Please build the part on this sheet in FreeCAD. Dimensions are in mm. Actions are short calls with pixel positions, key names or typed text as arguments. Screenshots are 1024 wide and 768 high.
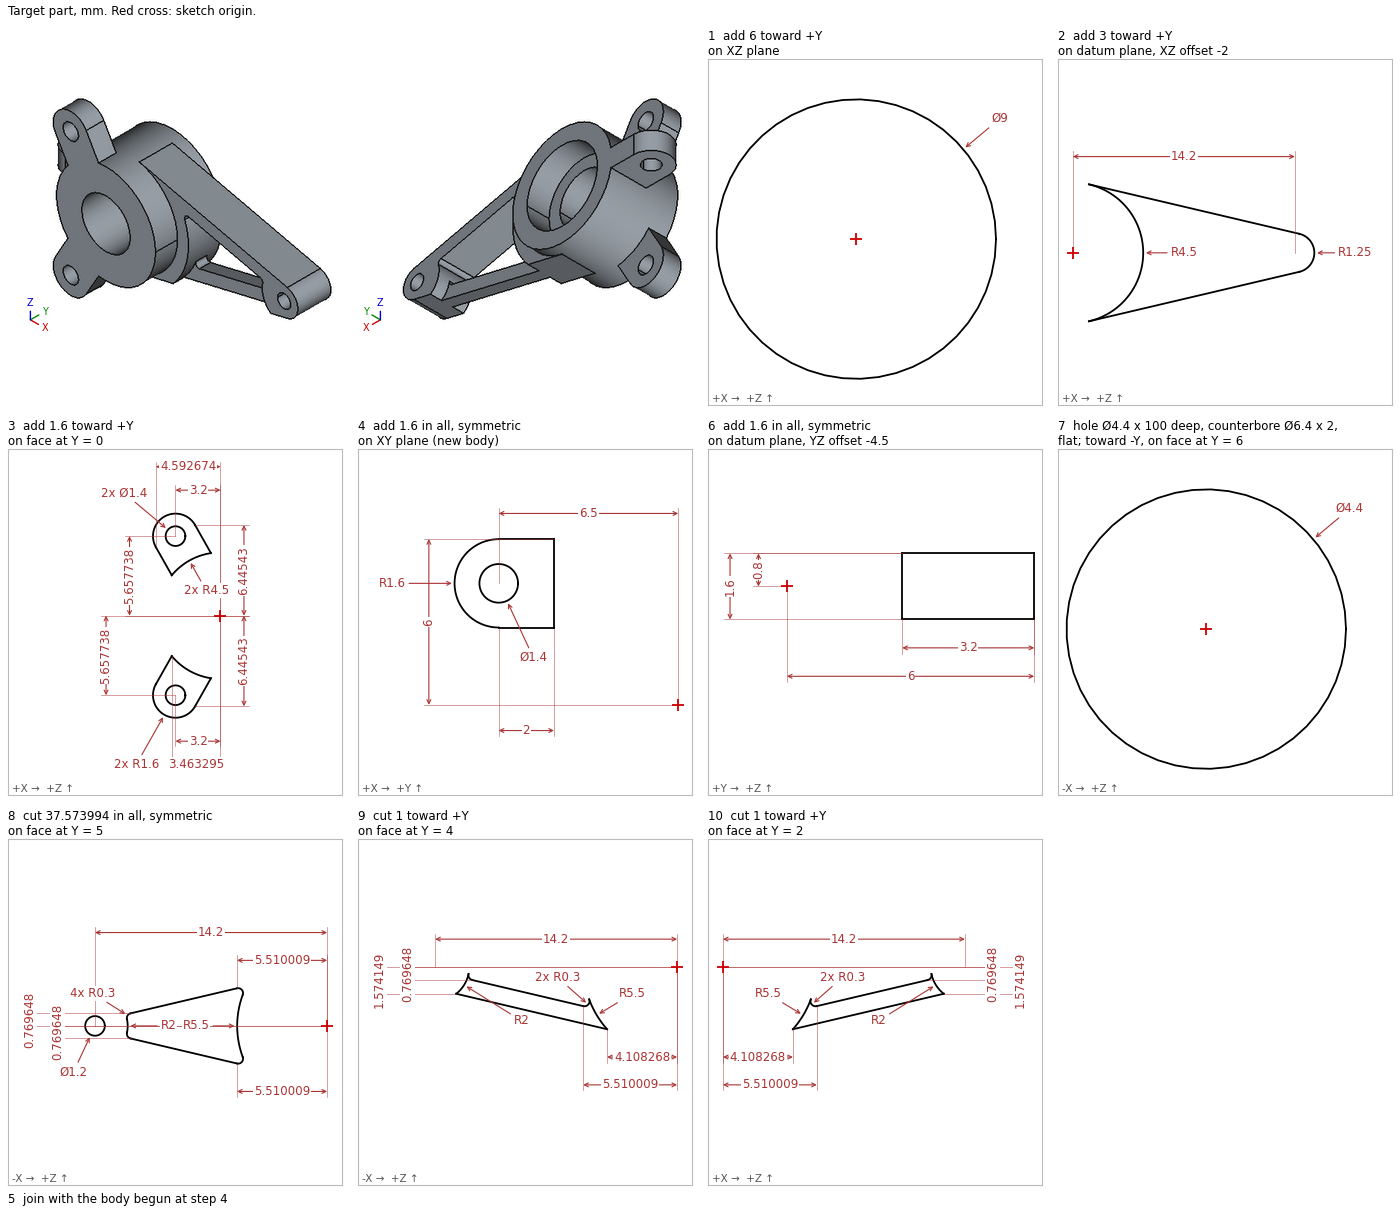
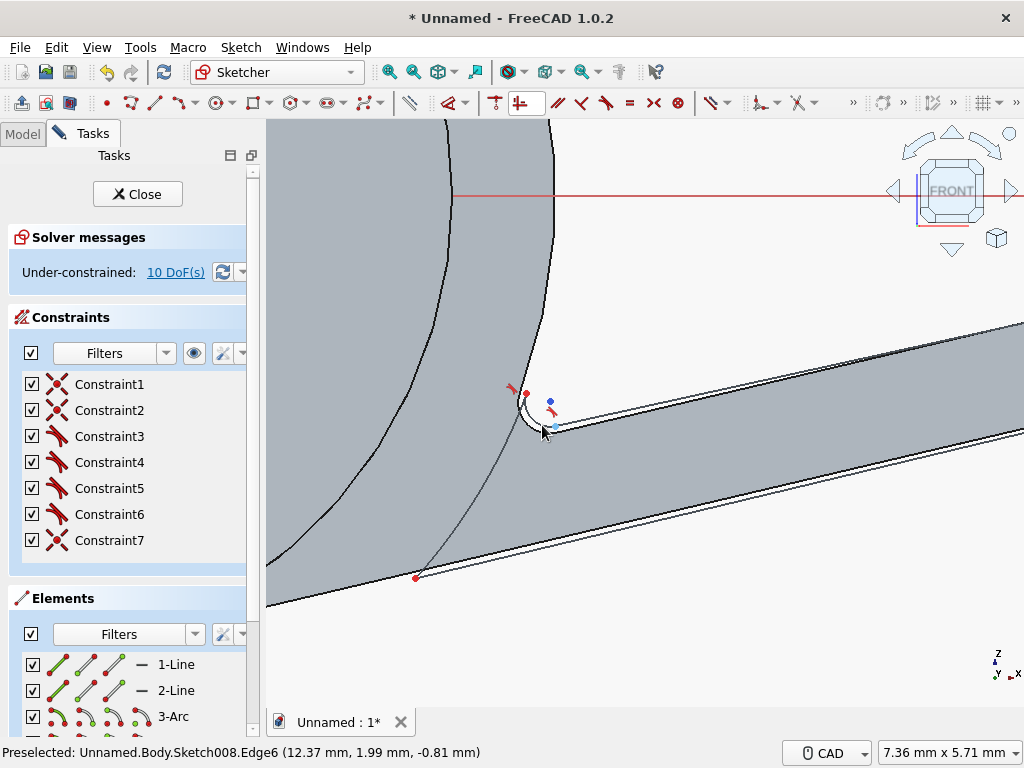
click(540, 425)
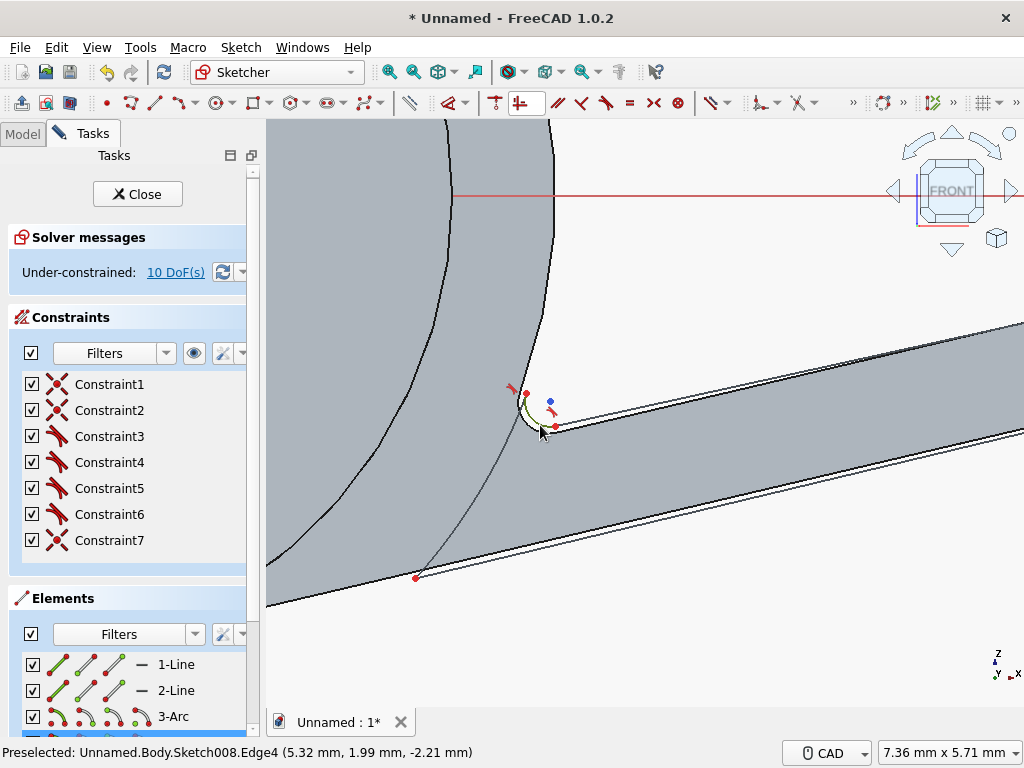
scroll(542, 425, down, 6)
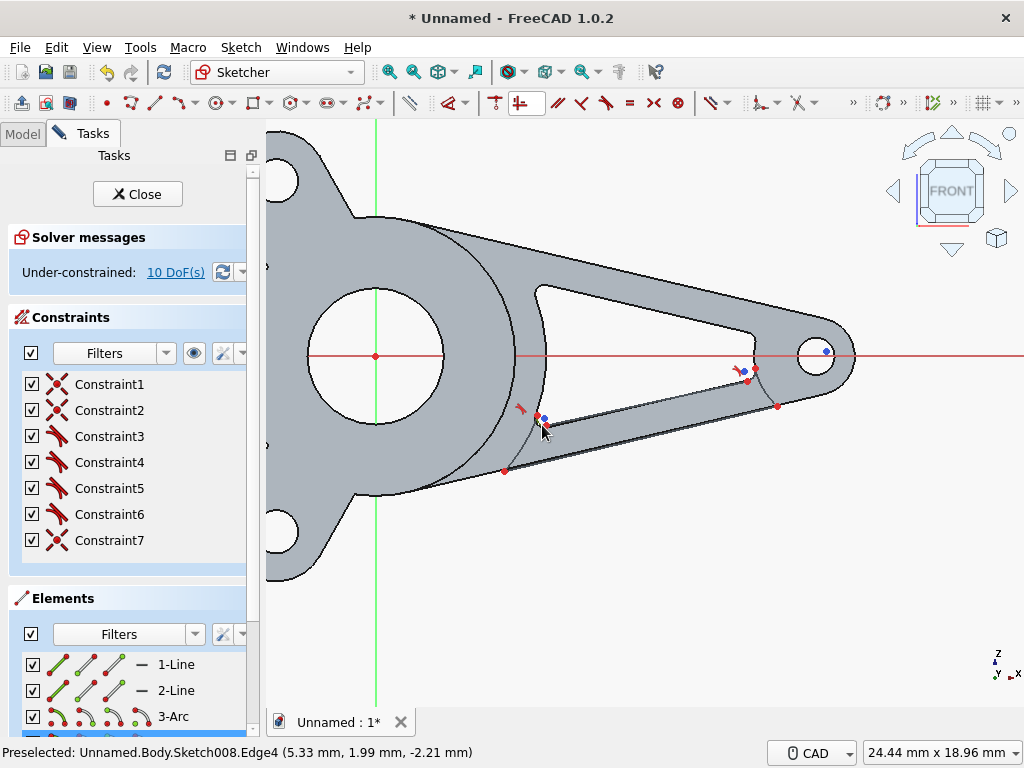
scroll(752, 379, up, 6)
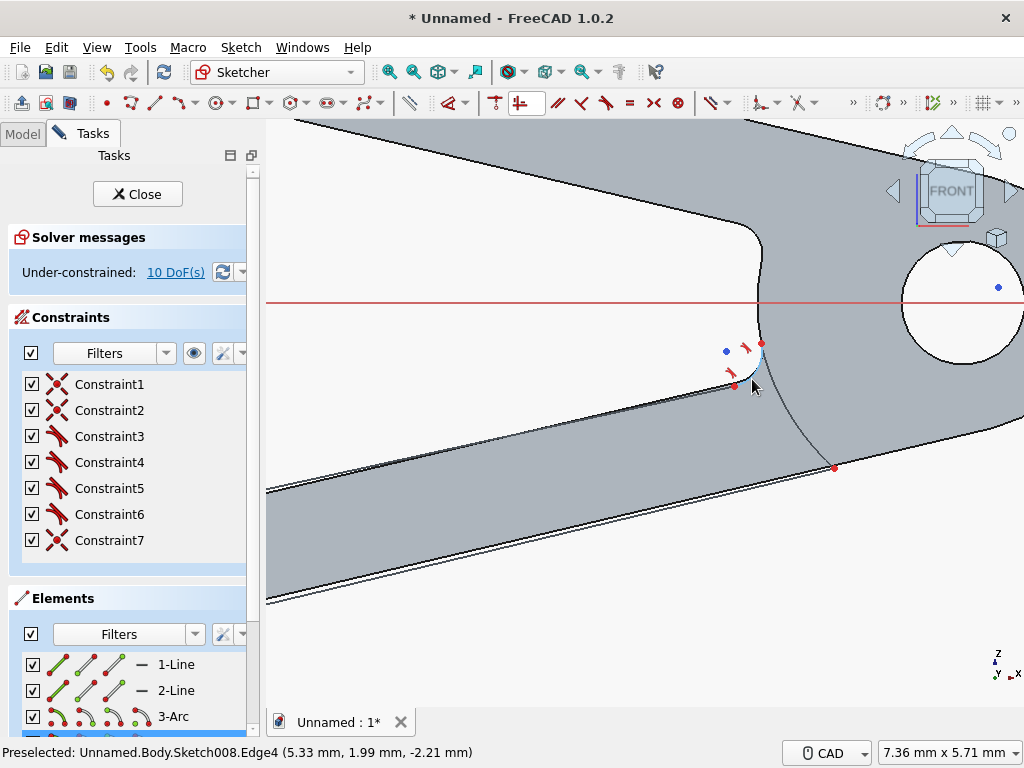
click(749, 379)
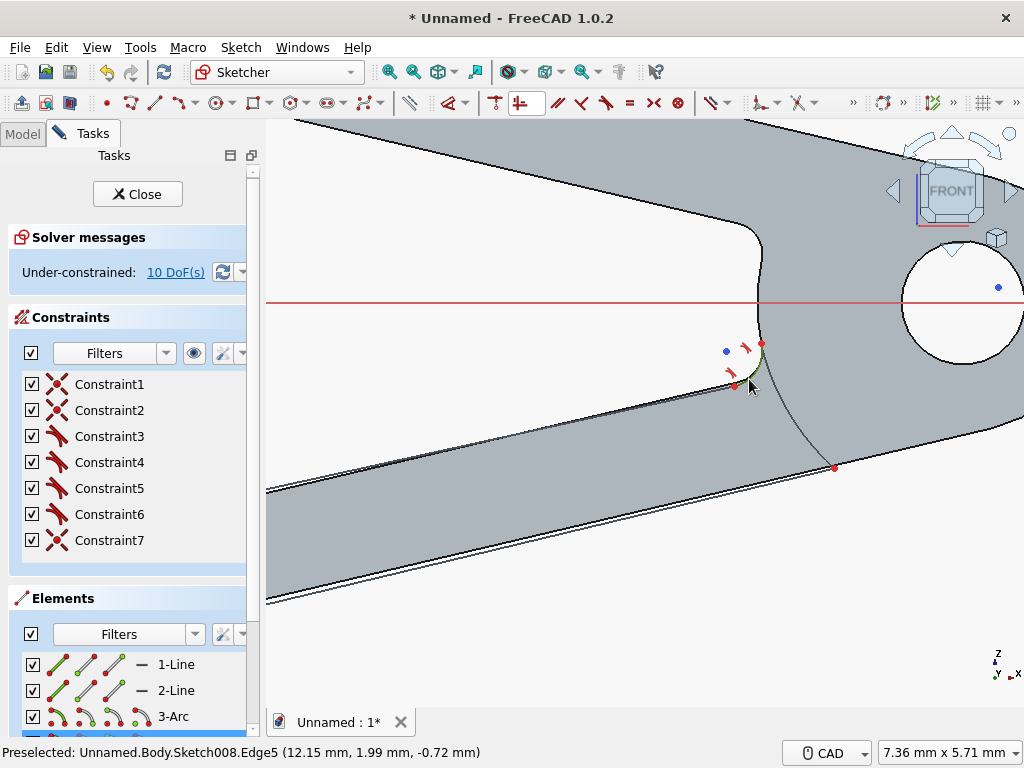
key(e)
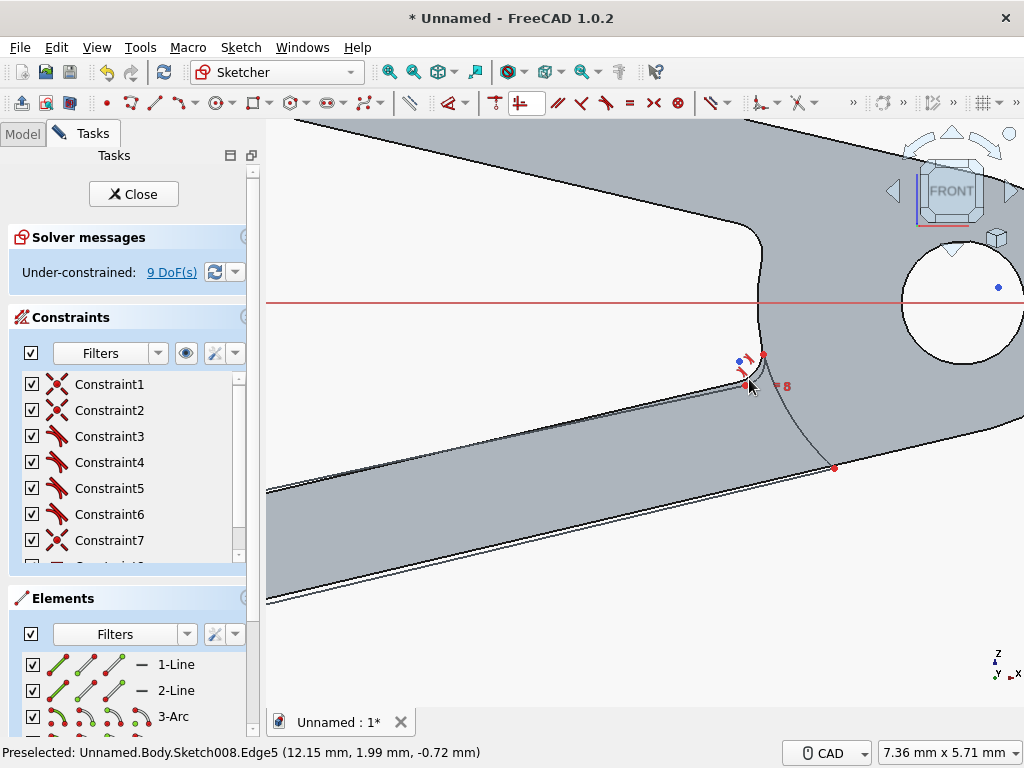
scroll(752, 379, down, 6)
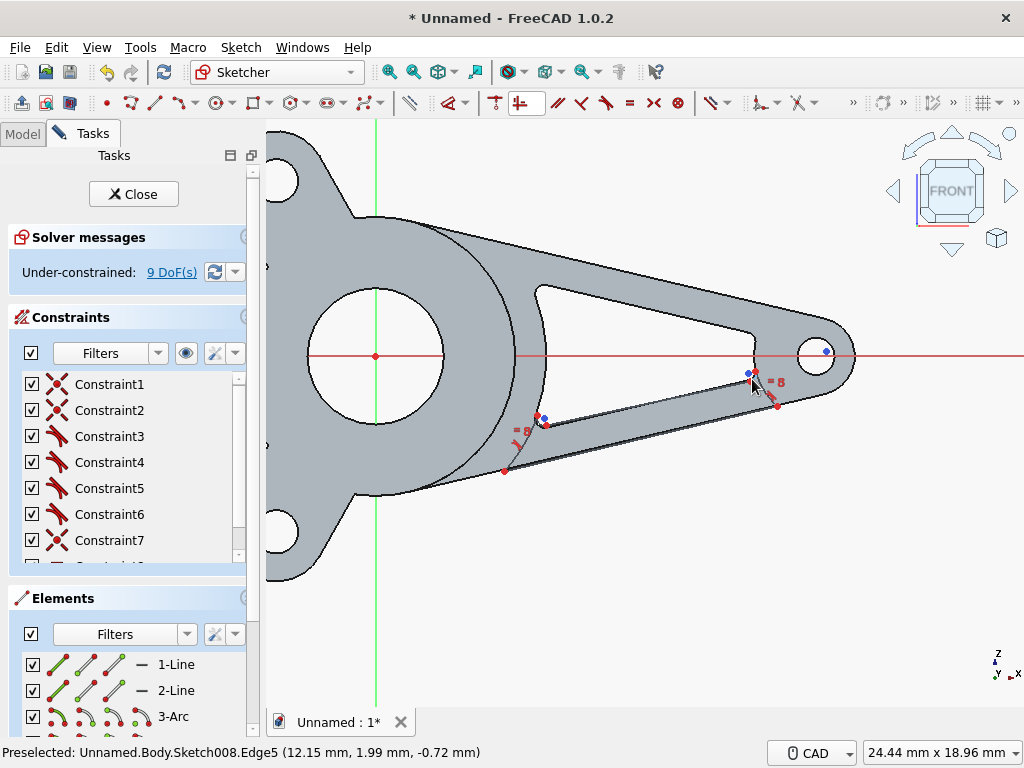
click(827, 352)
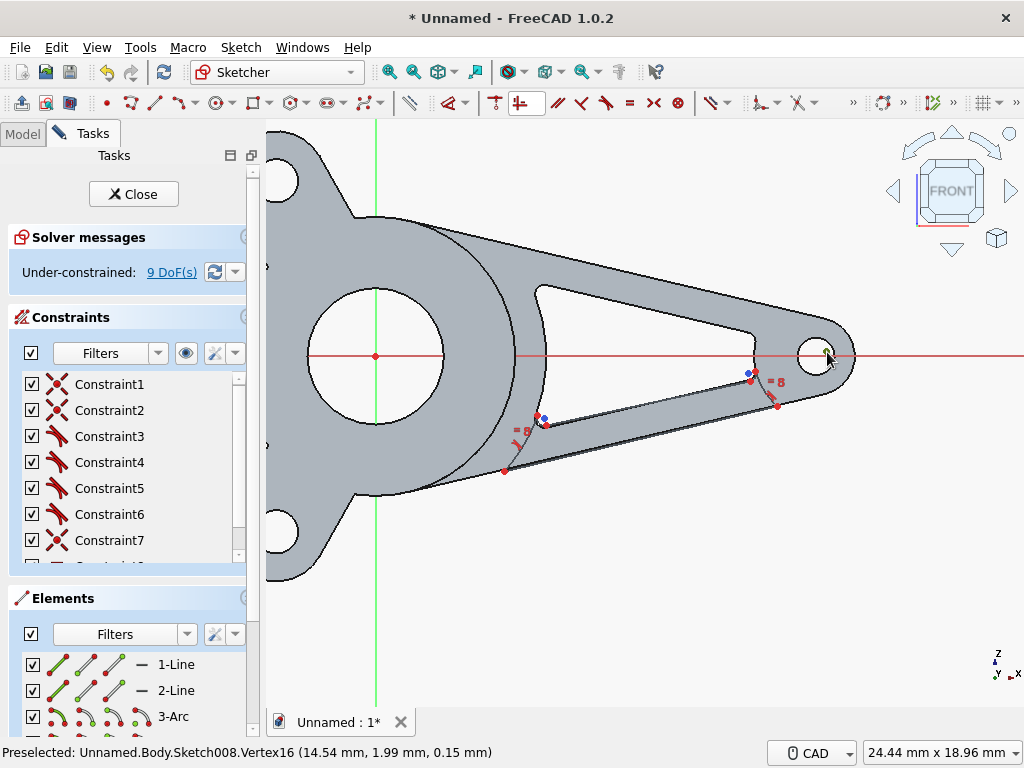
click(334, 356)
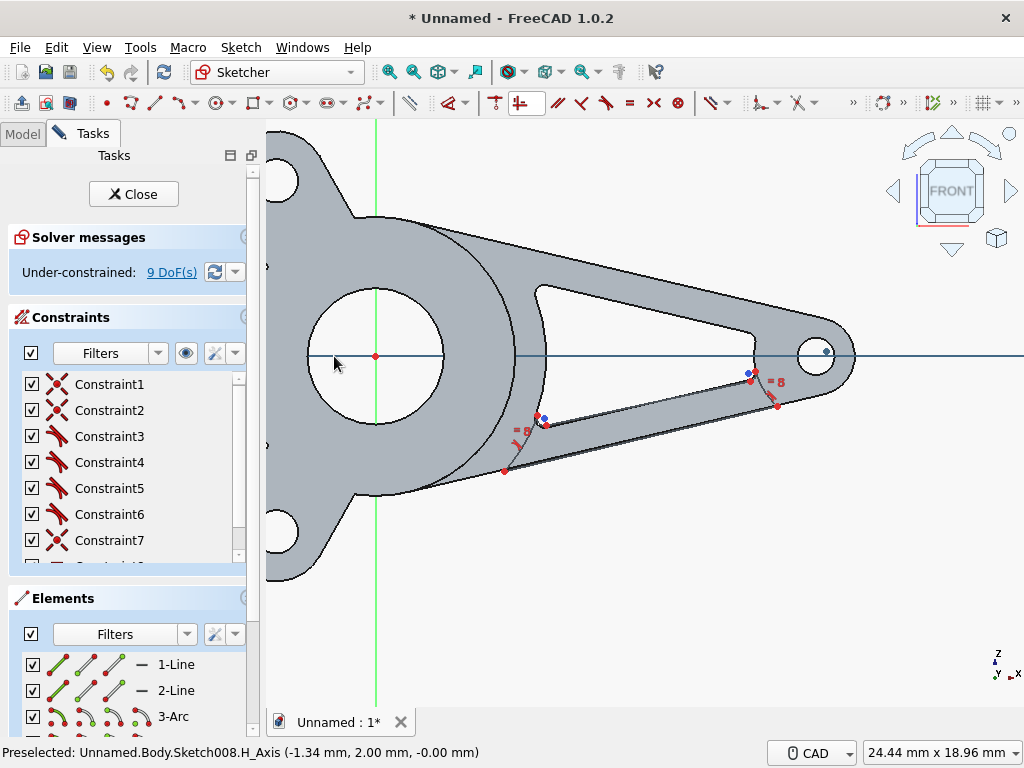
click(496, 104)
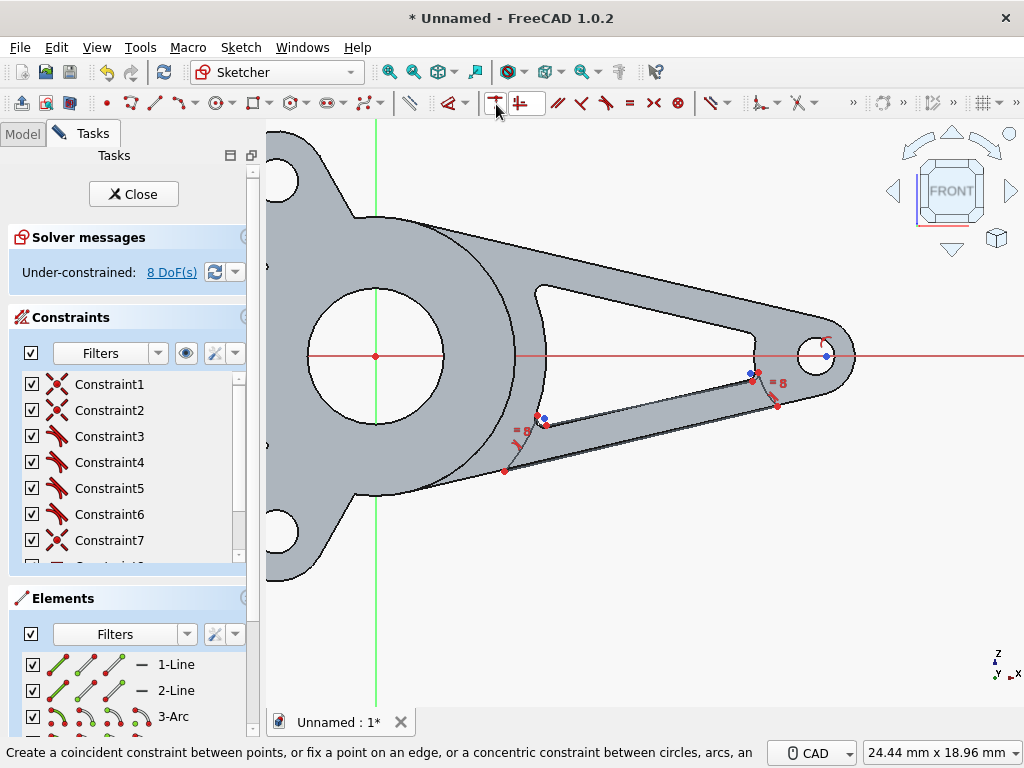
click(448, 104)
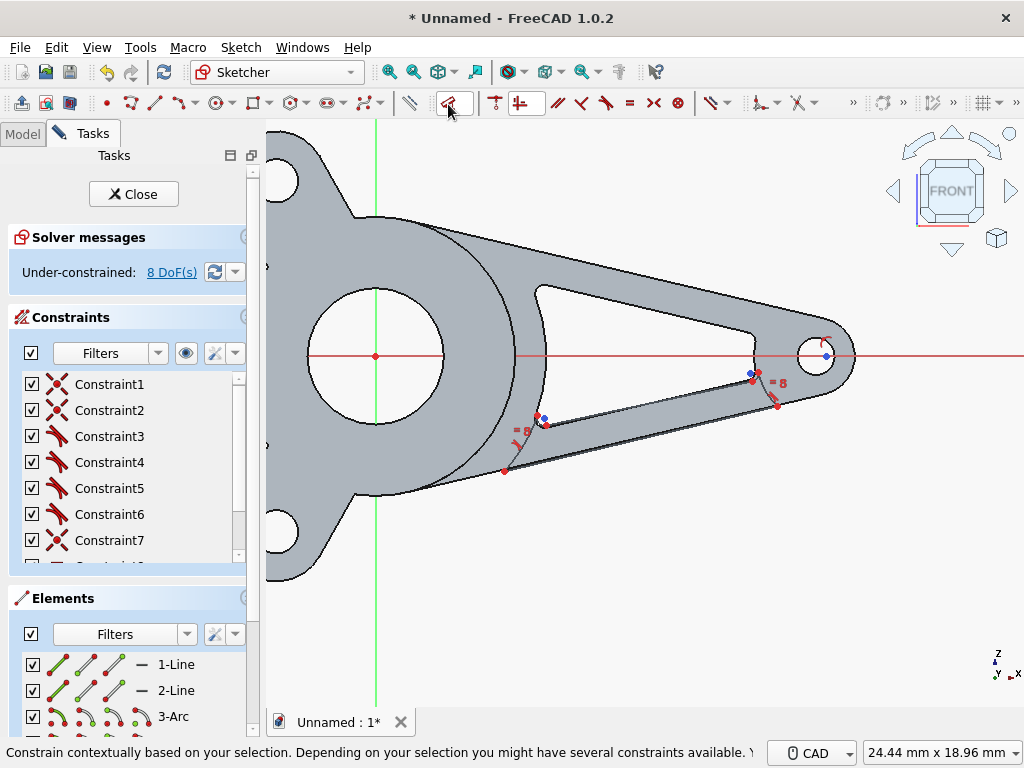
click(516, 456)
click(465, 540)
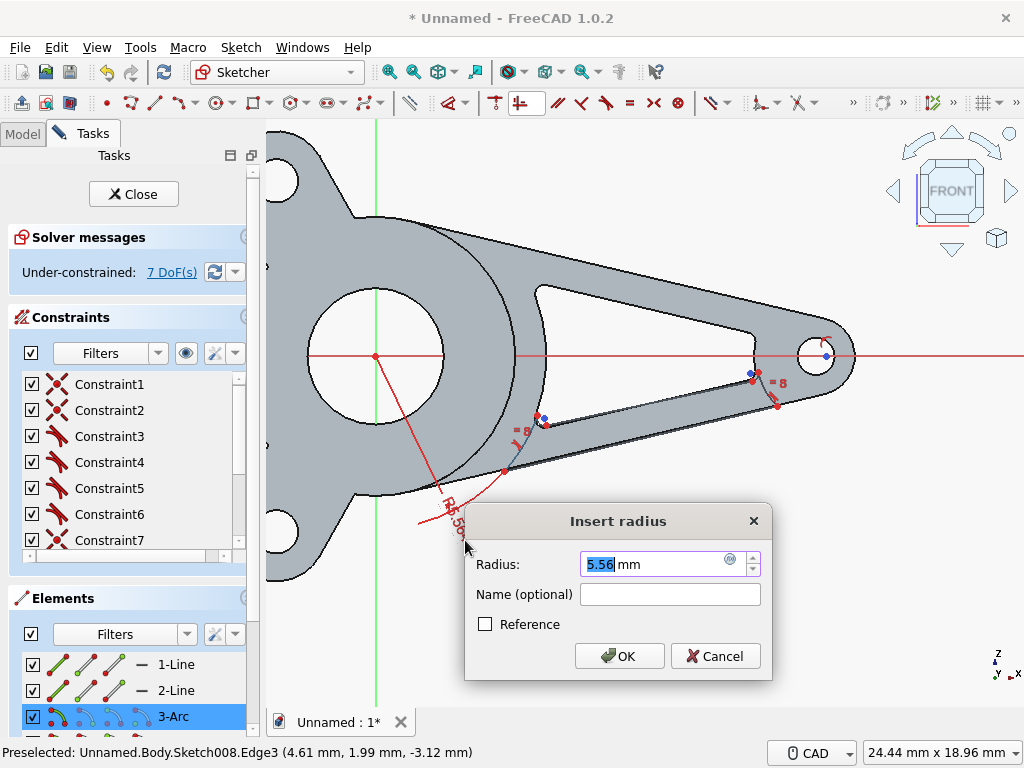
text(5.5)
key(Return)